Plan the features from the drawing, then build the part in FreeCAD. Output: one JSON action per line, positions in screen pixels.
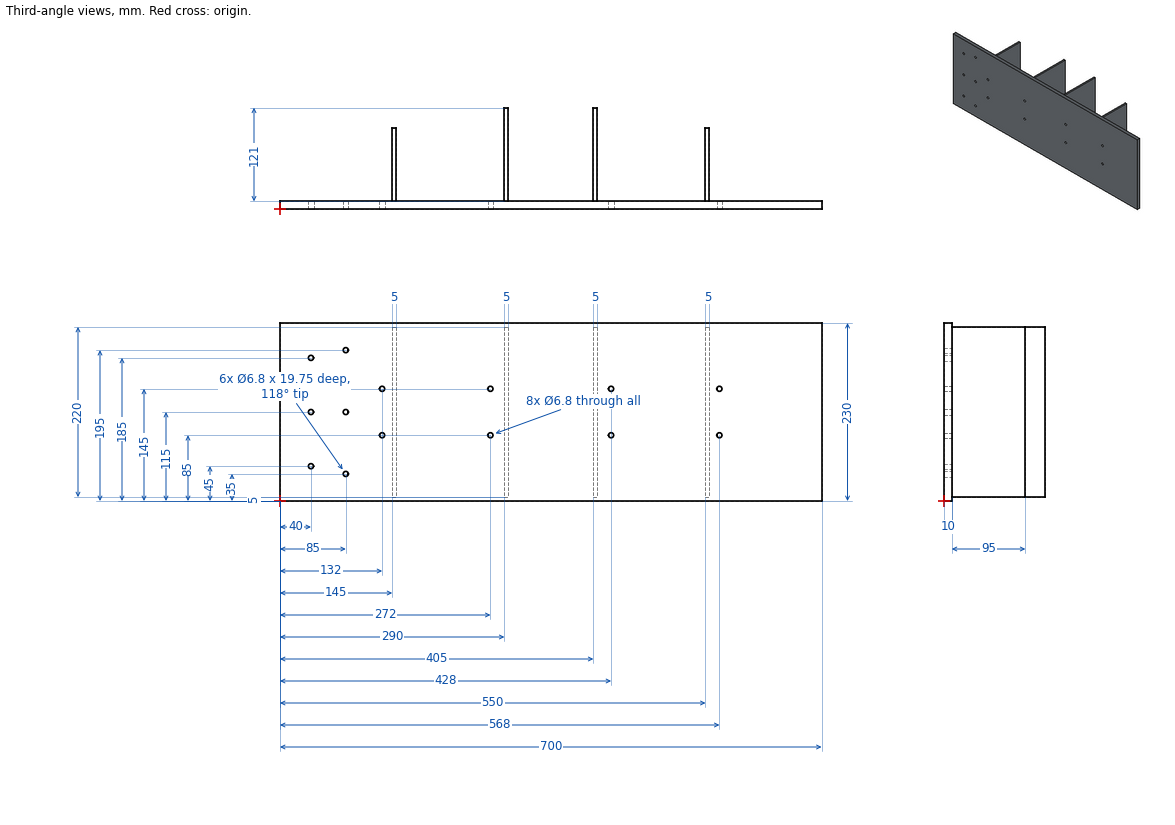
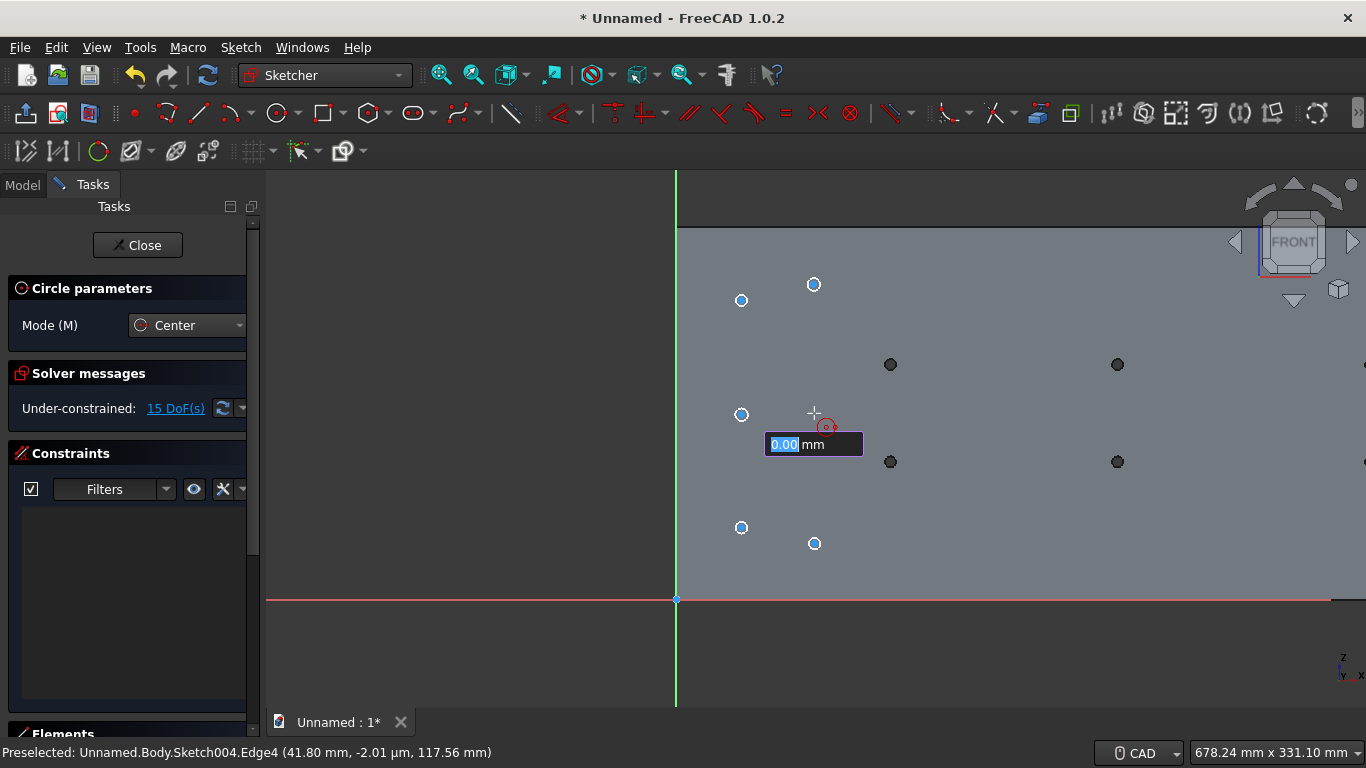
{"action": "scroll", "coordinate": [818, 409], "scroll_direction": "up", "scroll_amount": 6}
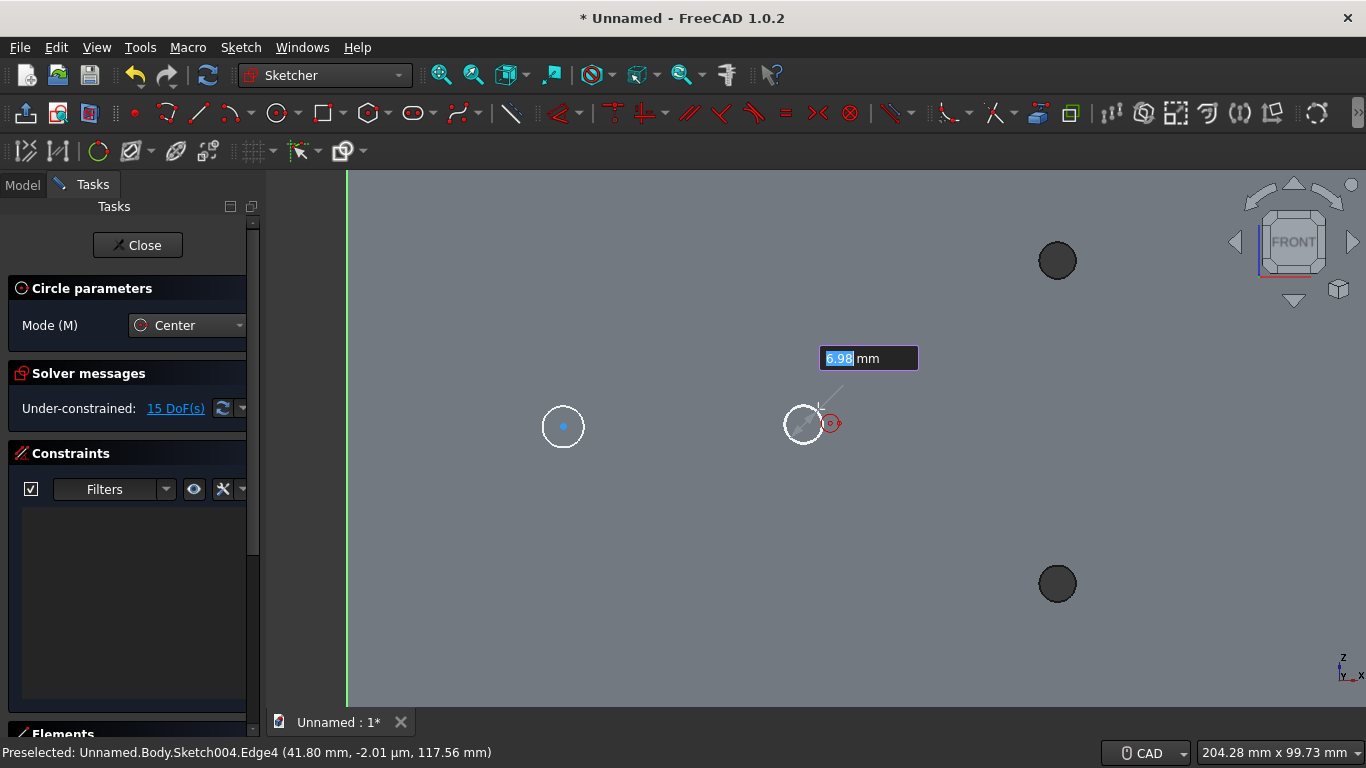
{"action": "left_click", "coordinate": [817, 409]}
{"action": "key", "text": "Escape"}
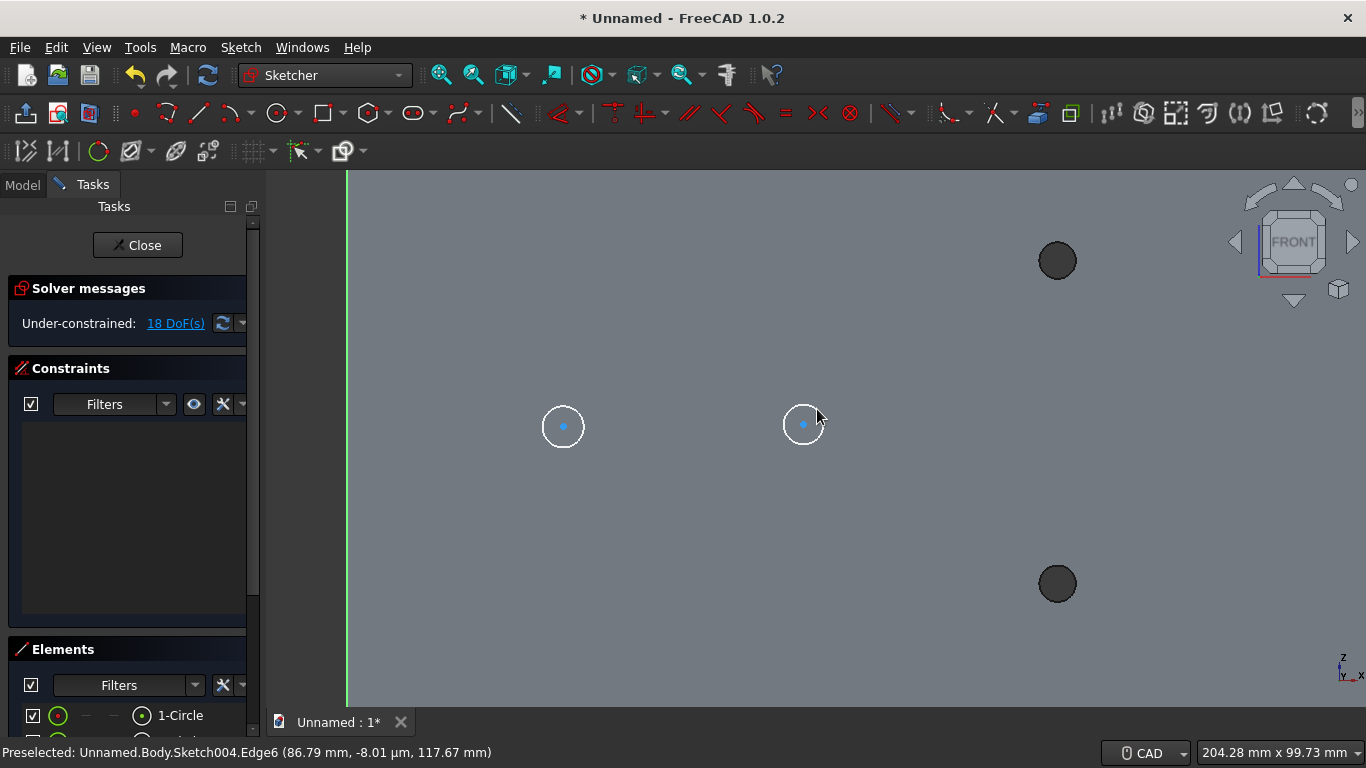
{"action": "scroll", "coordinate": [818, 409], "scroll_direction": "down", "scroll_amount": 6}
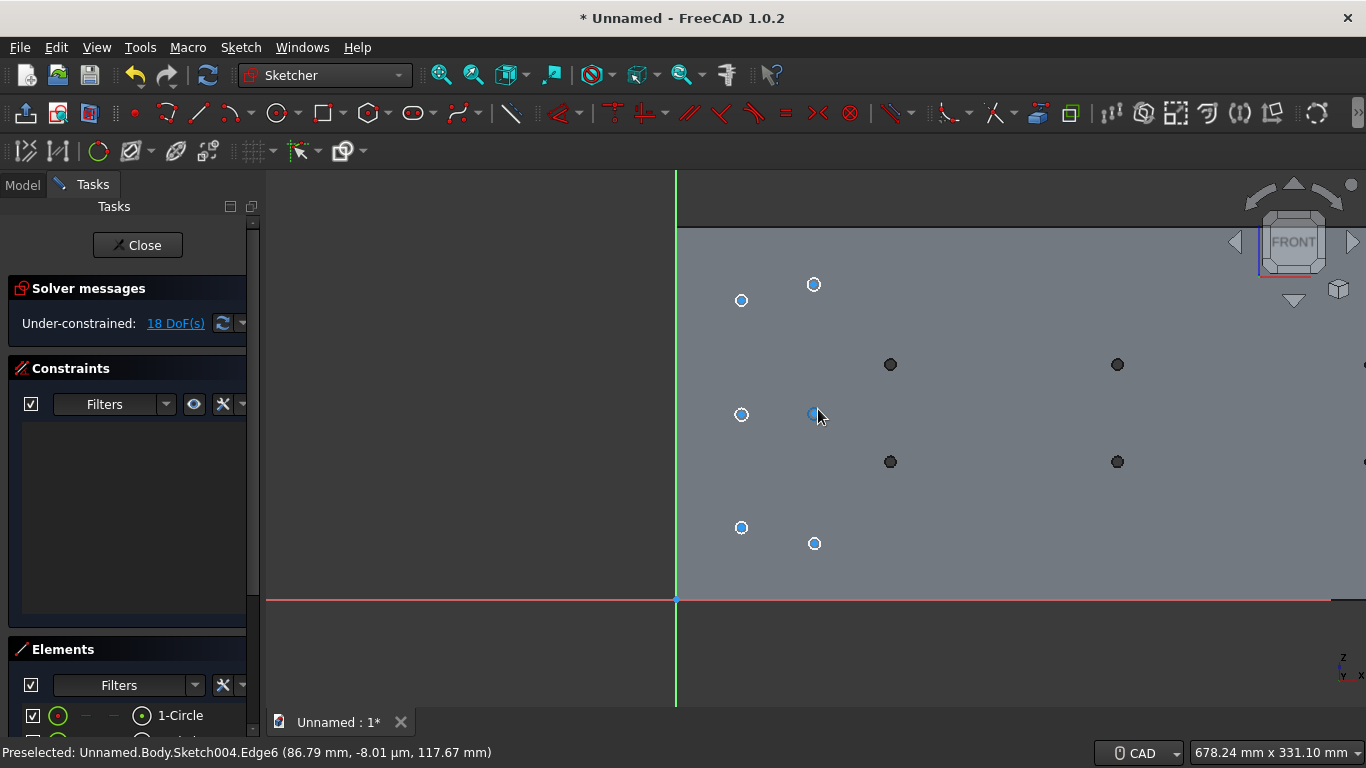
{"action": "scroll", "coordinate": [819, 540], "scroll_direction": "up", "scroll_amount": 5}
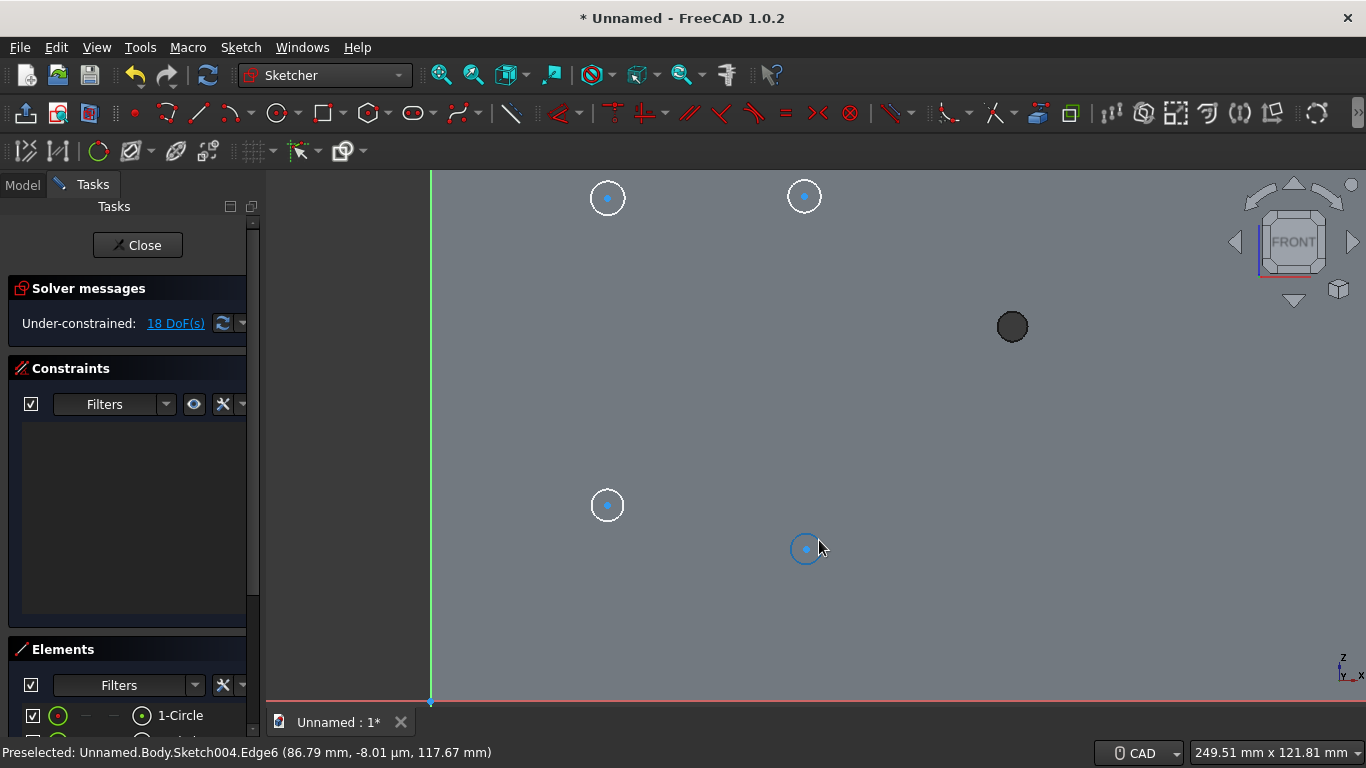
{"action": "left_click", "coordinate": [817, 538]}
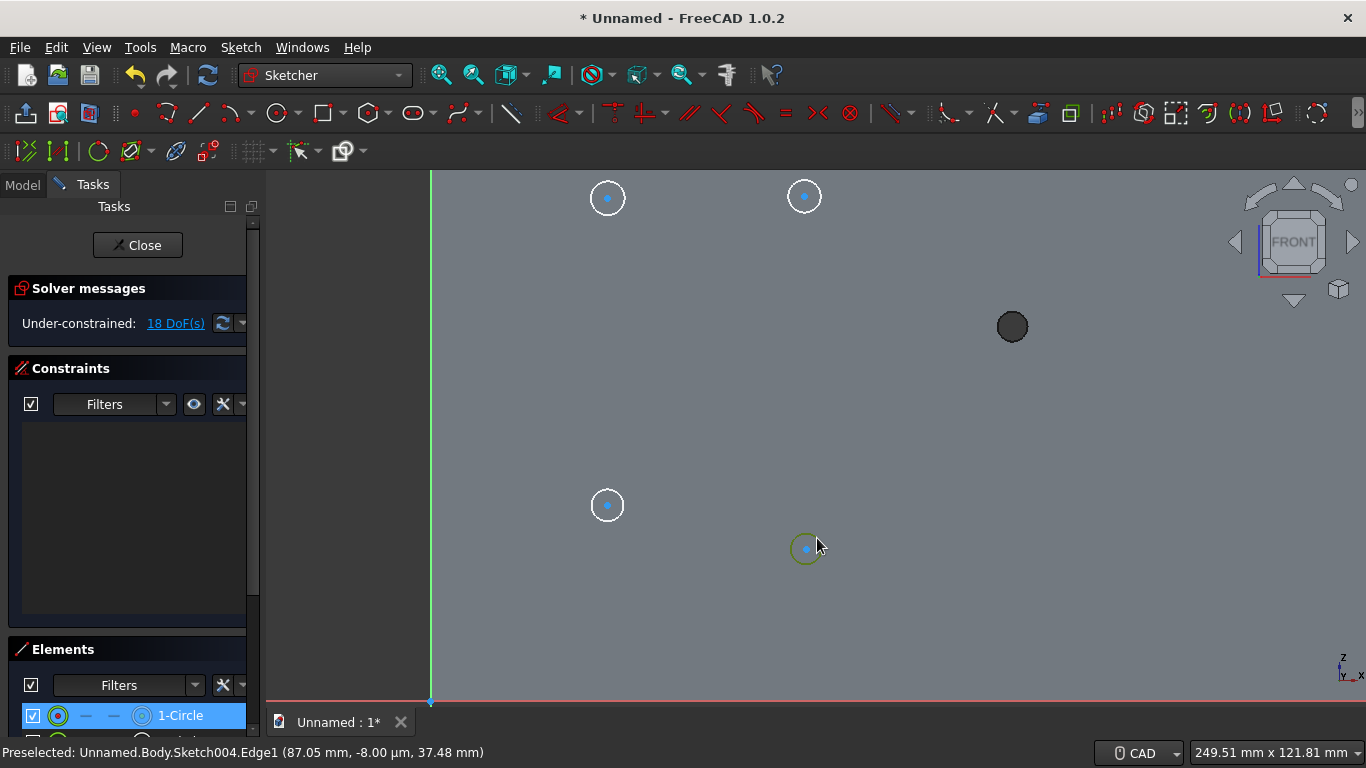
{"action": "left_click", "coordinate": [619, 494]}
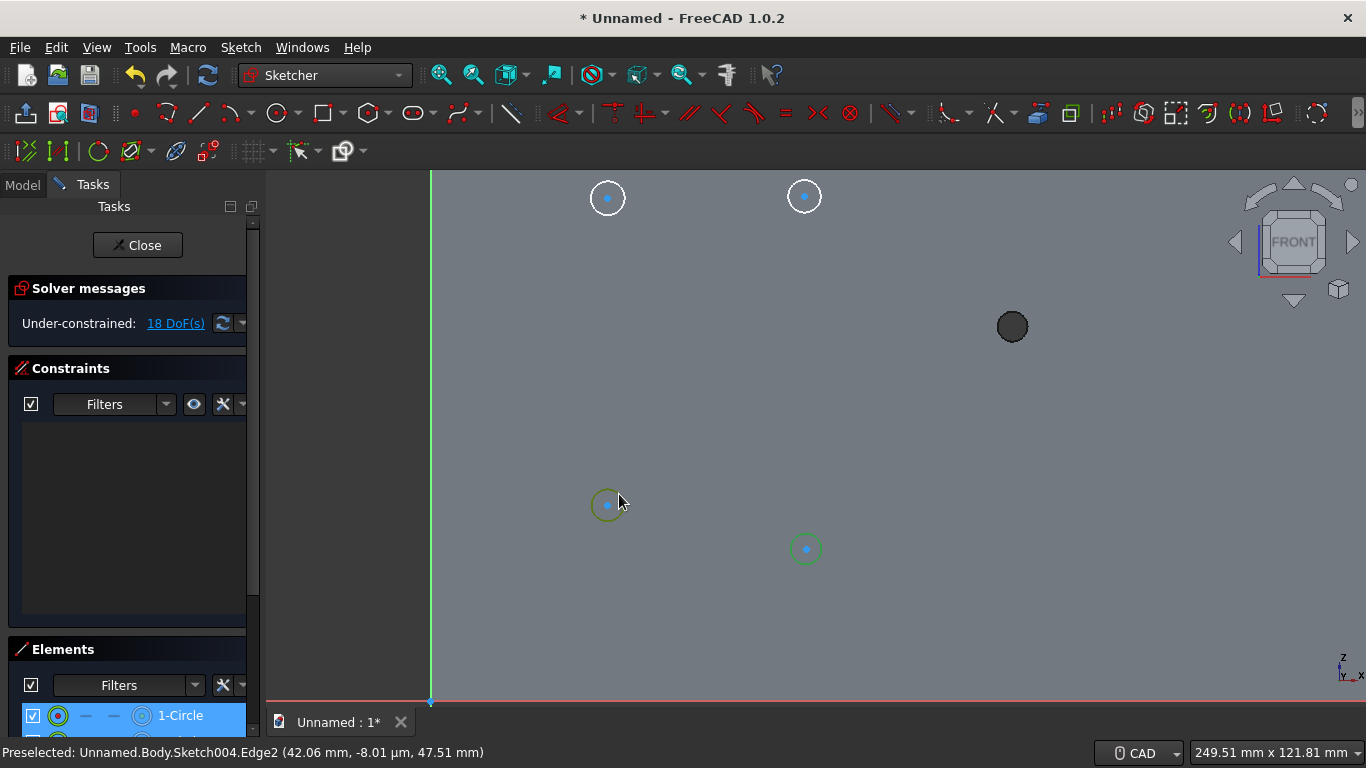
{"action": "scroll", "coordinate": [819, 540], "scroll_direction": "down", "scroll_amount": 5}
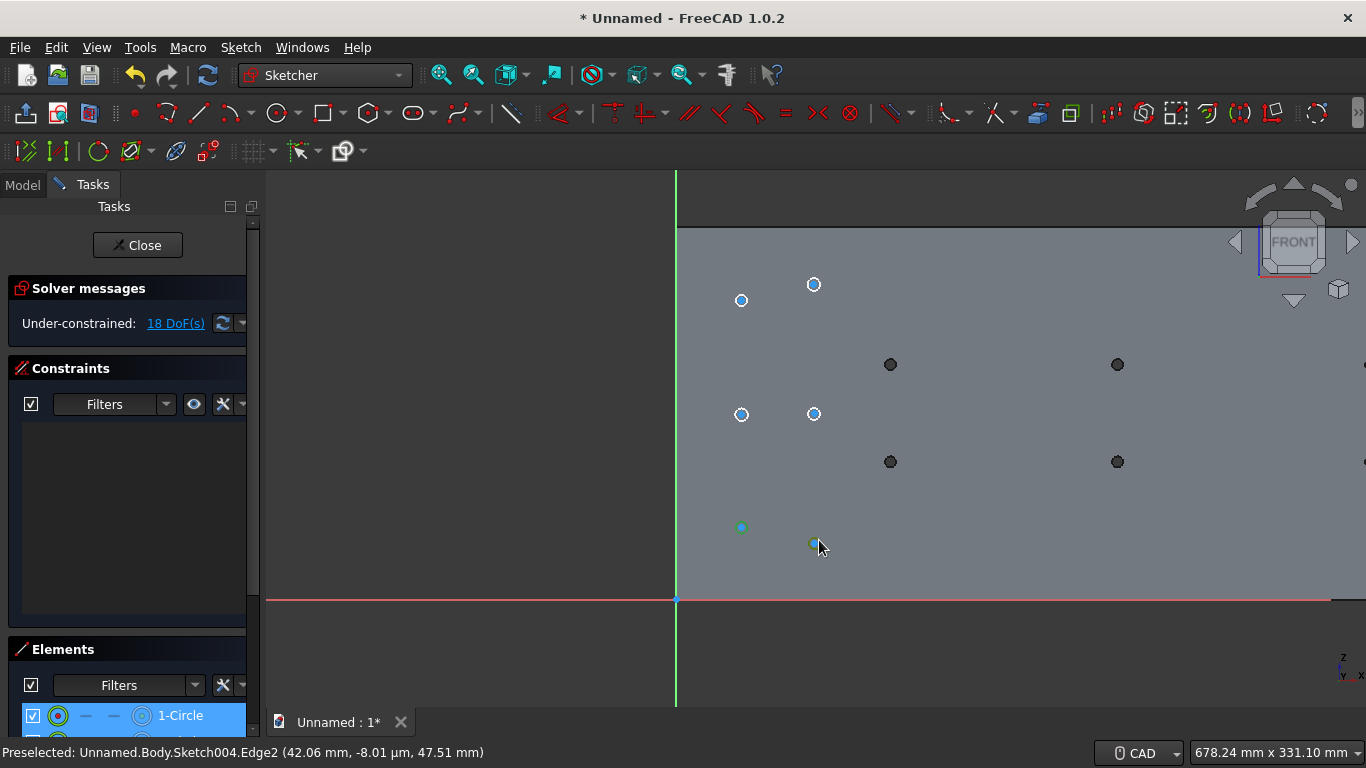
{"action": "scroll", "coordinate": [745, 296], "scroll_direction": "up", "scroll_amount": 5}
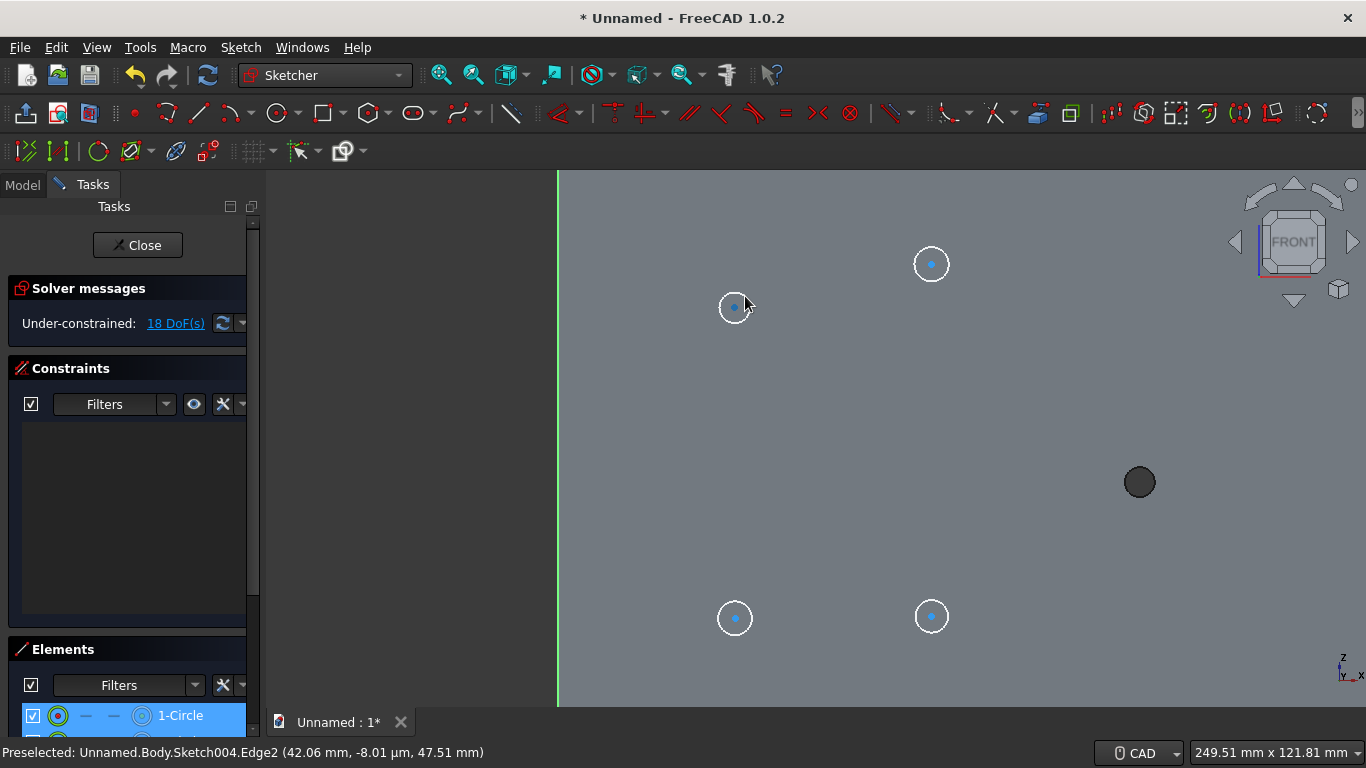
{"action": "left_click", "coordinate": [746, 297]}